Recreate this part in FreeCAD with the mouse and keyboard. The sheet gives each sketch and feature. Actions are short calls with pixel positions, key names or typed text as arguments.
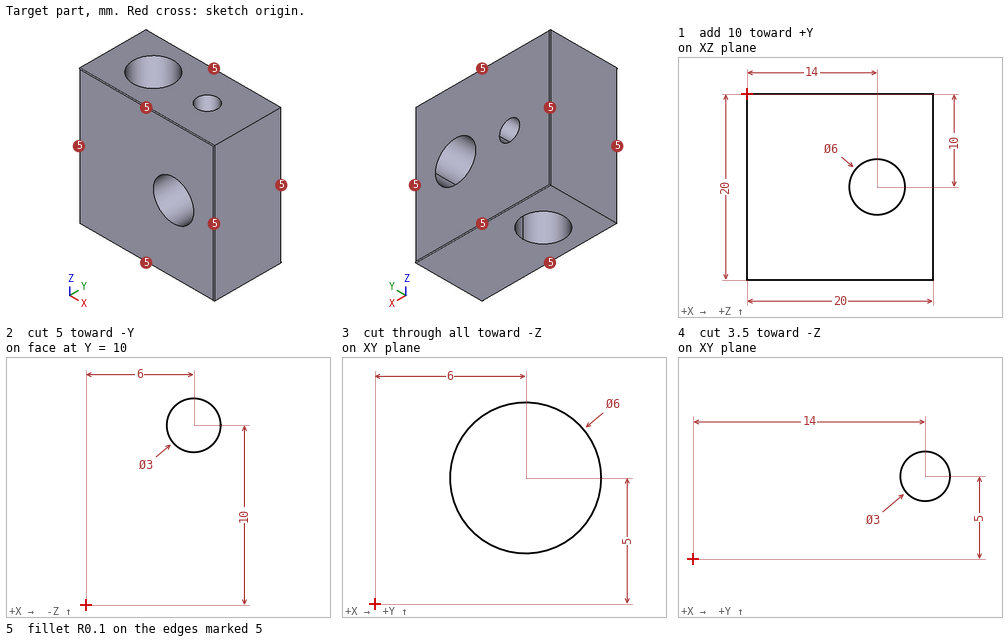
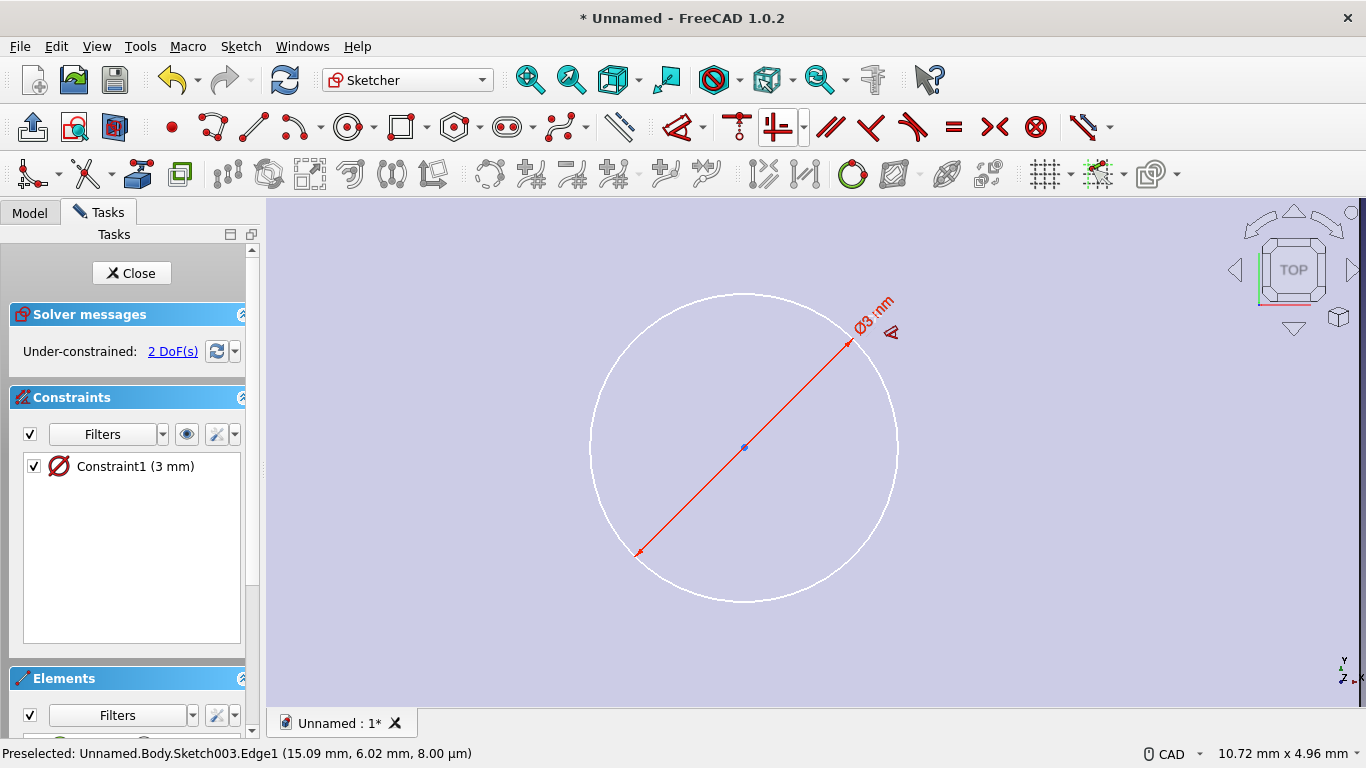
click(744, 448)
click(778, 564)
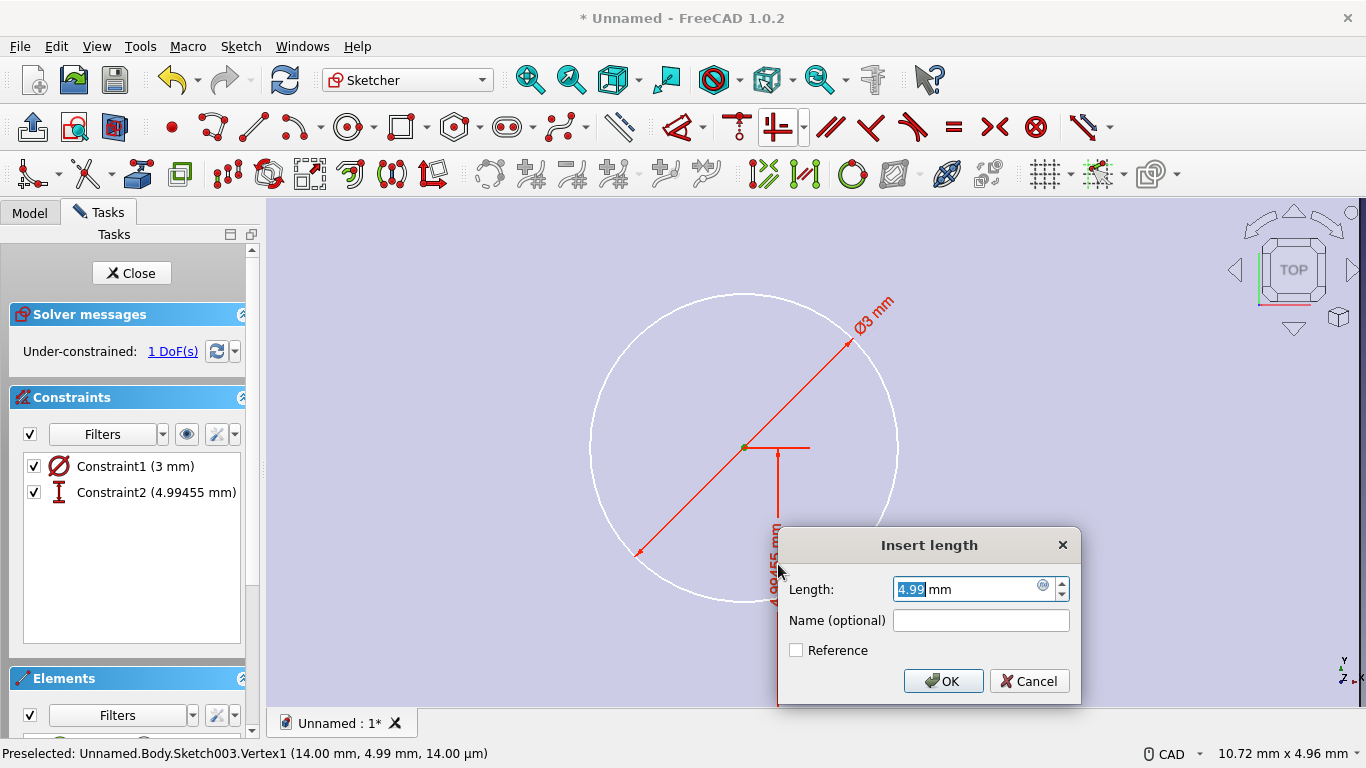
text(5)
key(Return)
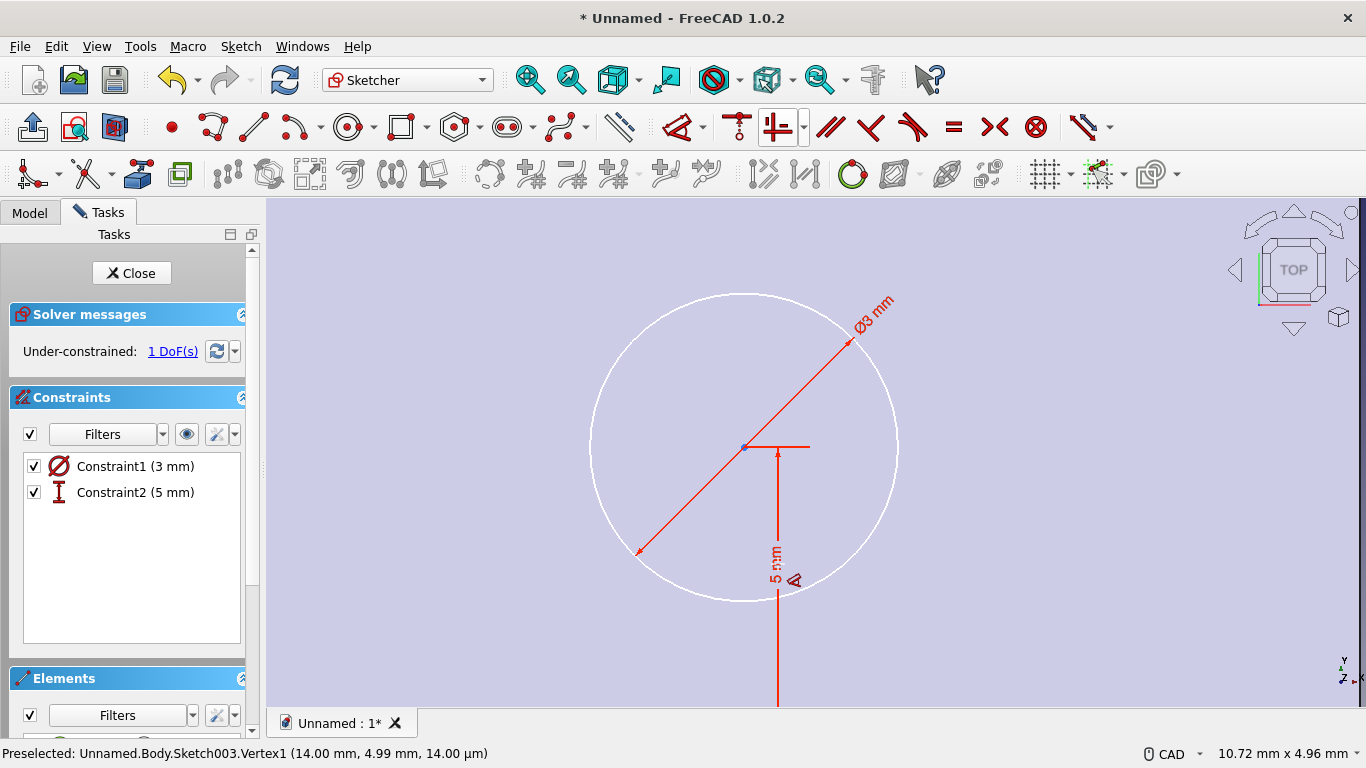
click(744, 447)
click(519, 413)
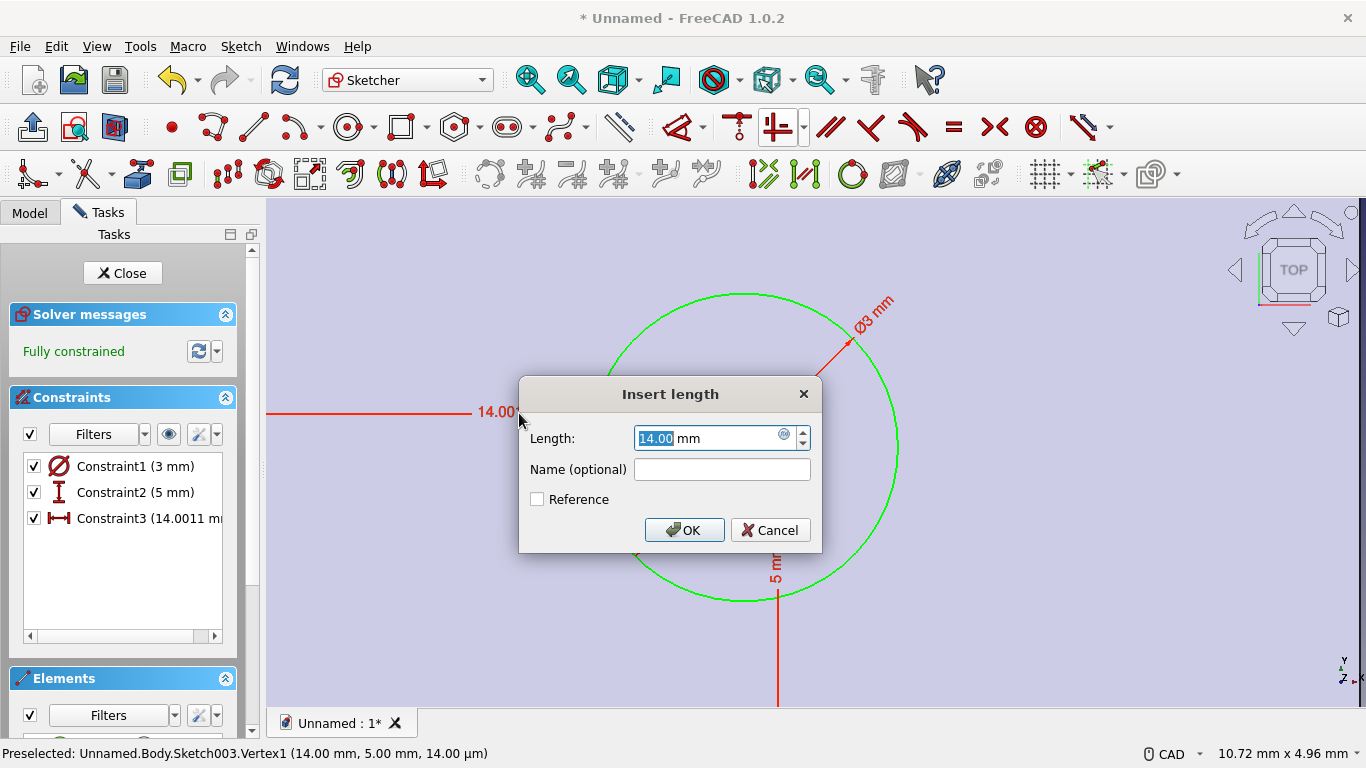
text(14)
key(Return)
key(Escape)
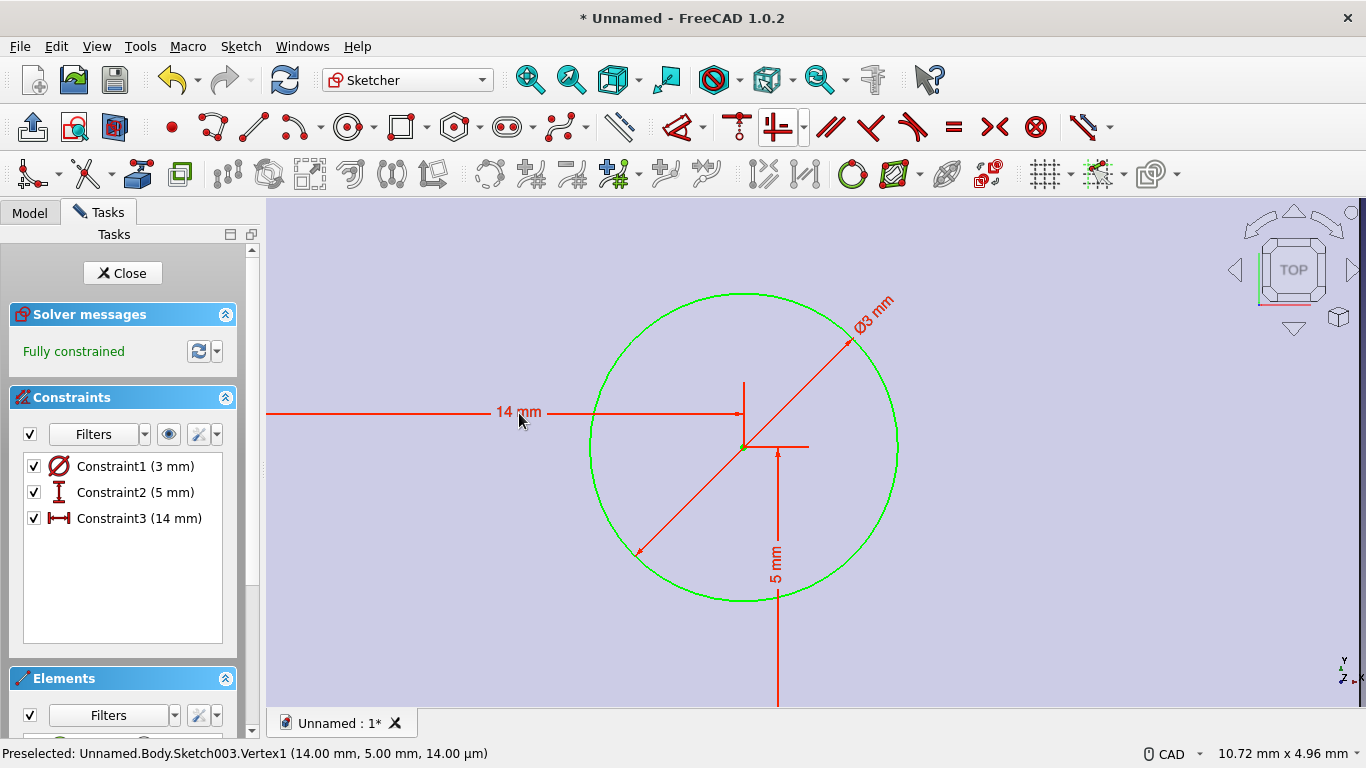
click(123, 273)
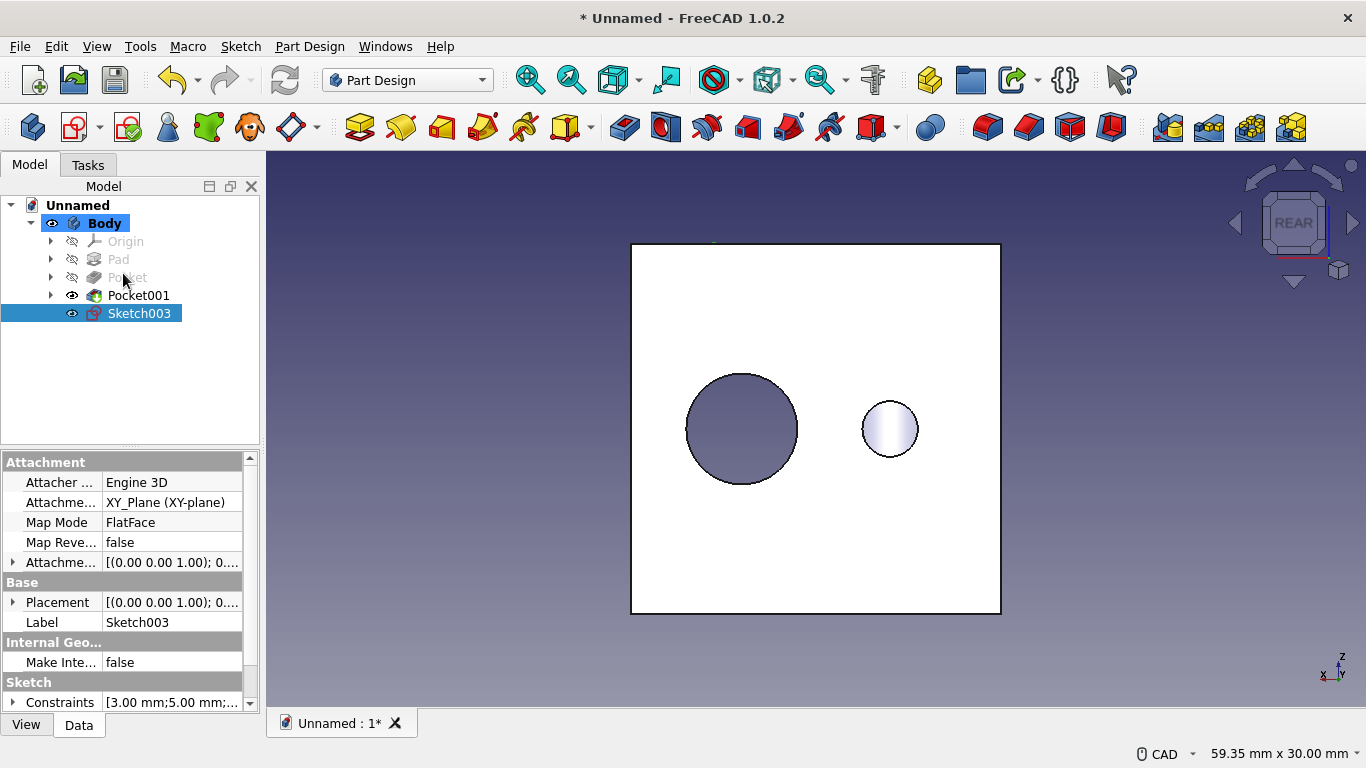
click(625, 128)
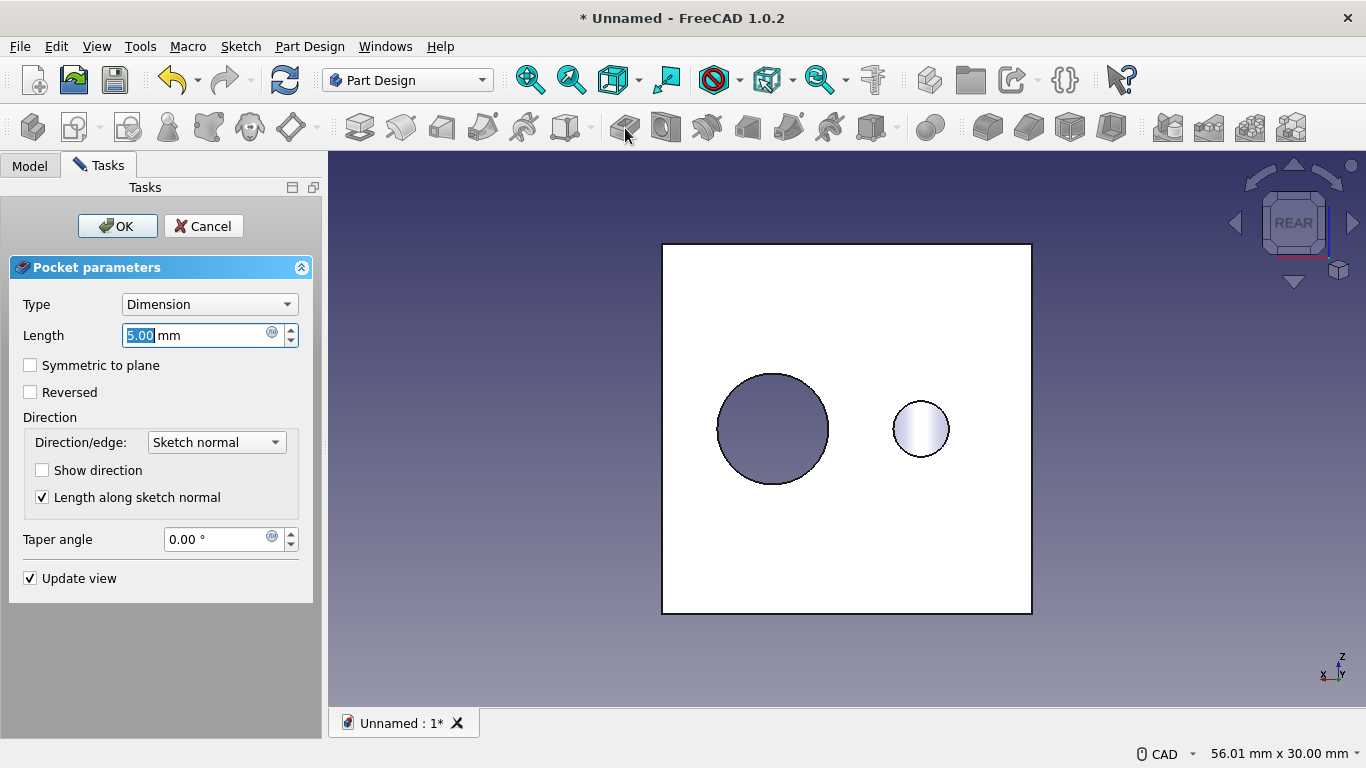
text(3.5)
key(Tab)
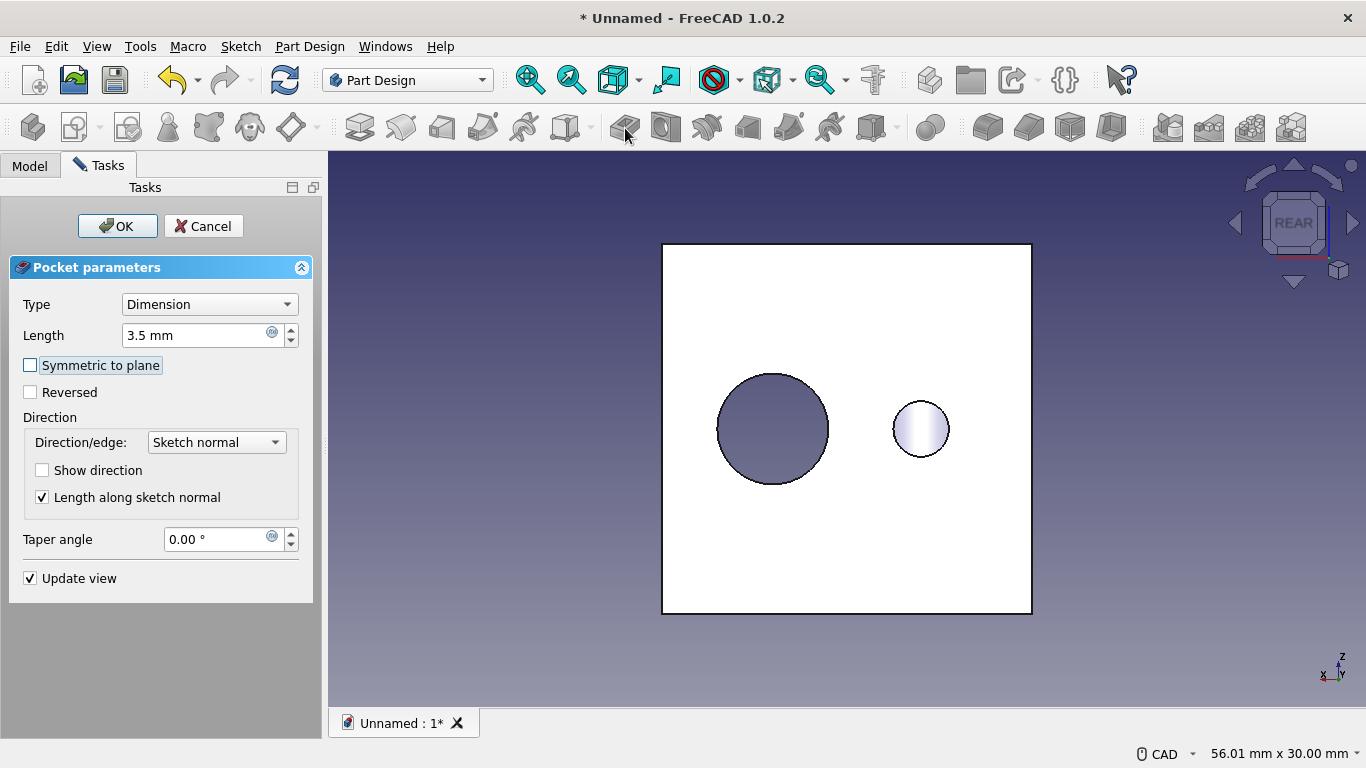
click(118, 226)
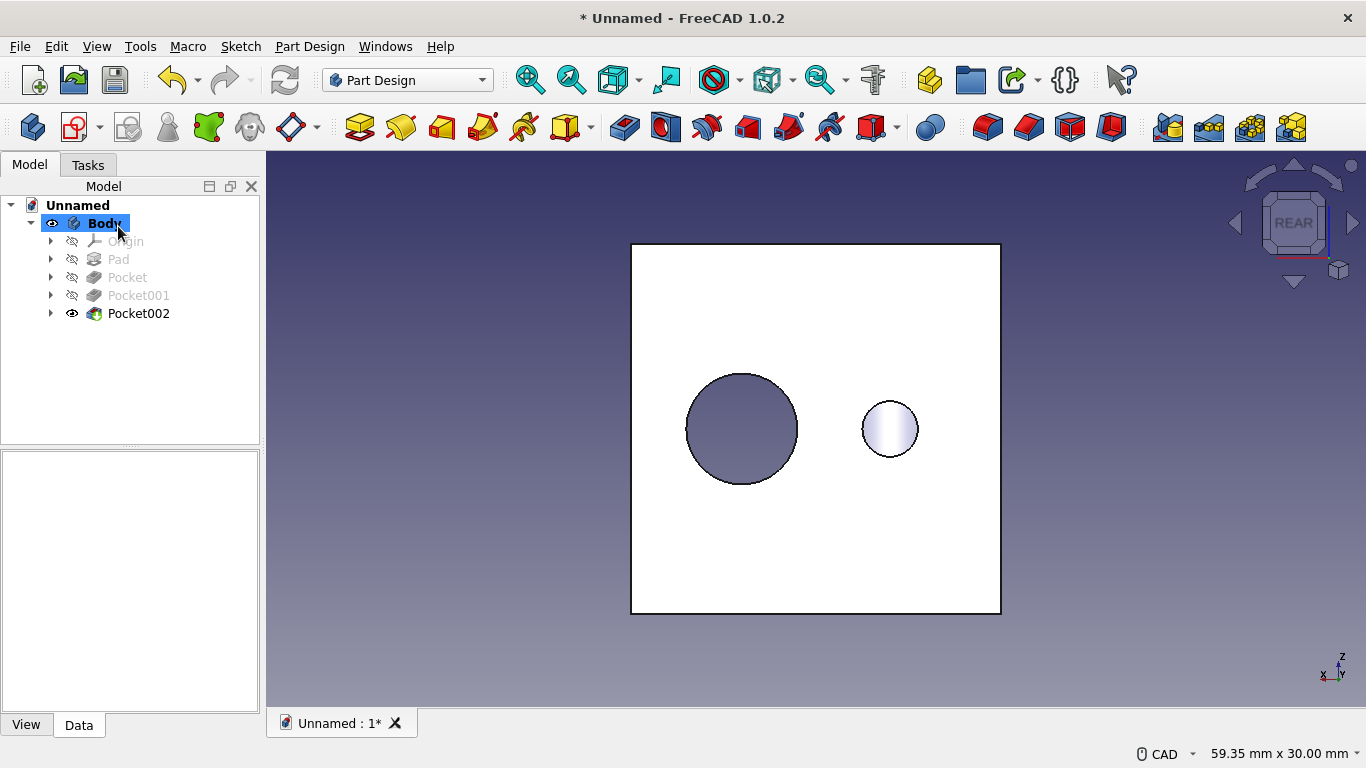
click(816, 613)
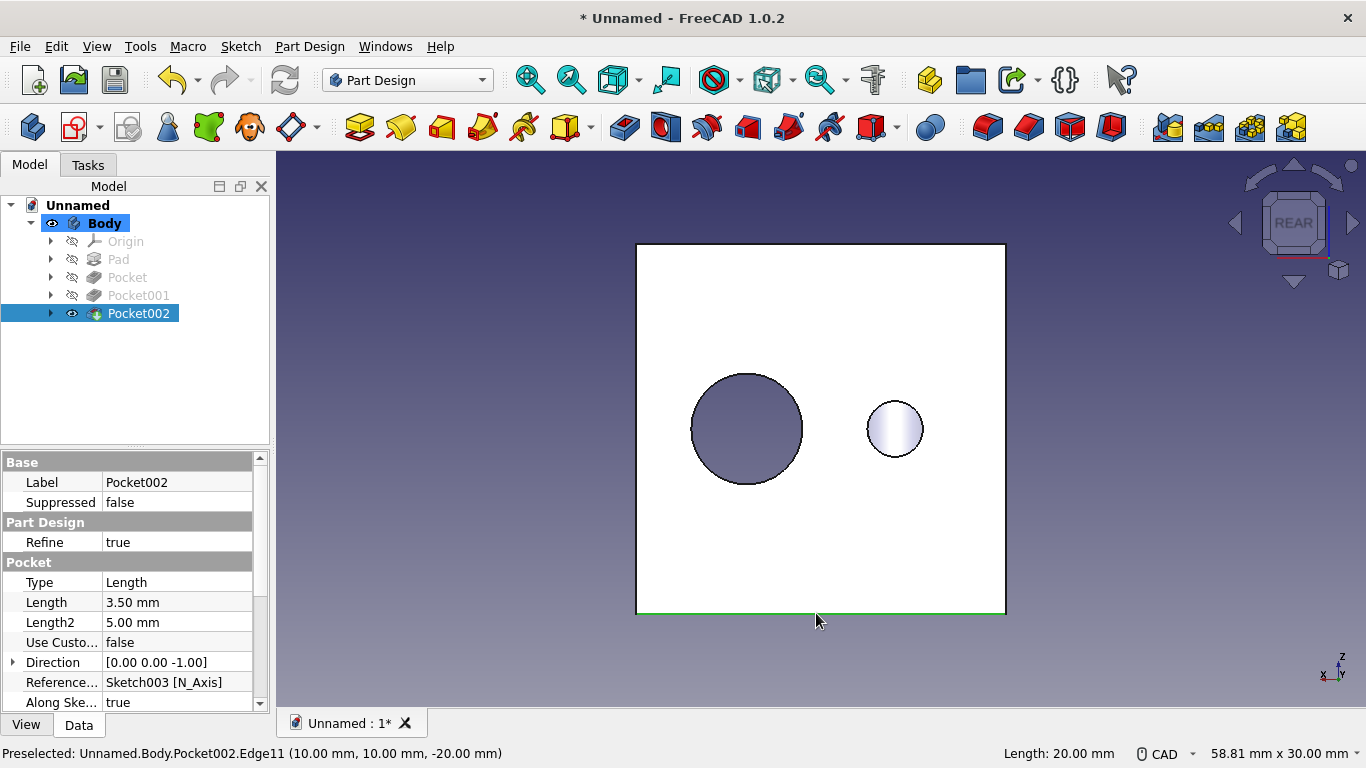
click(1006, 428, ctrl)